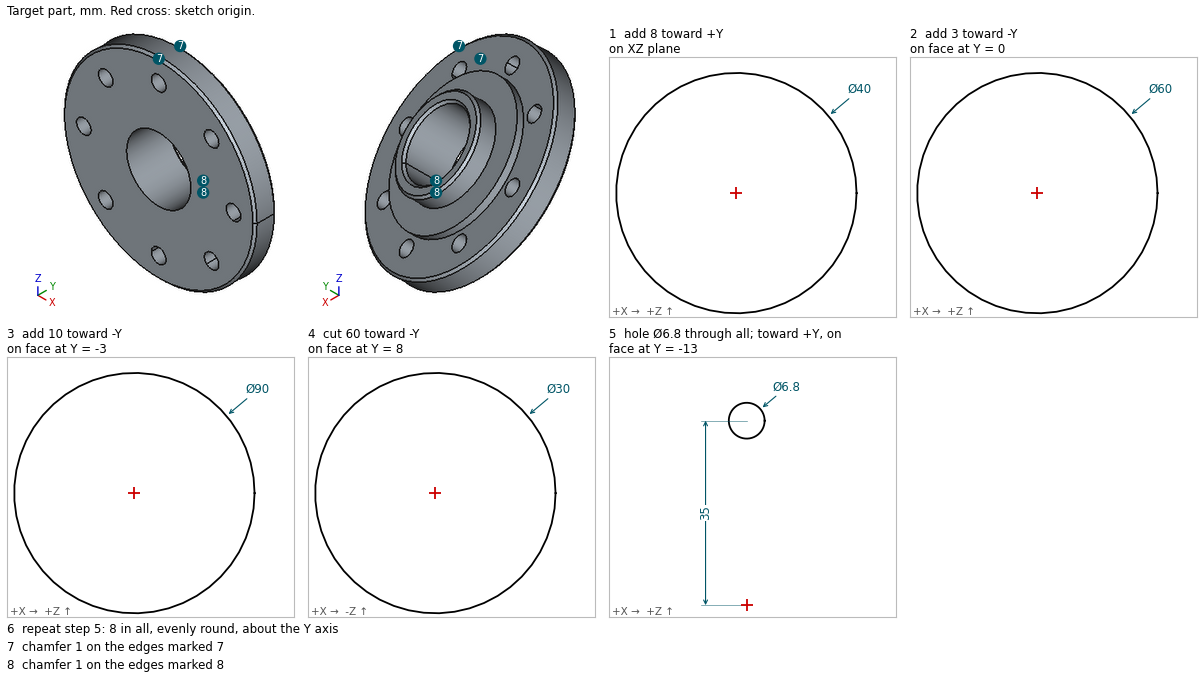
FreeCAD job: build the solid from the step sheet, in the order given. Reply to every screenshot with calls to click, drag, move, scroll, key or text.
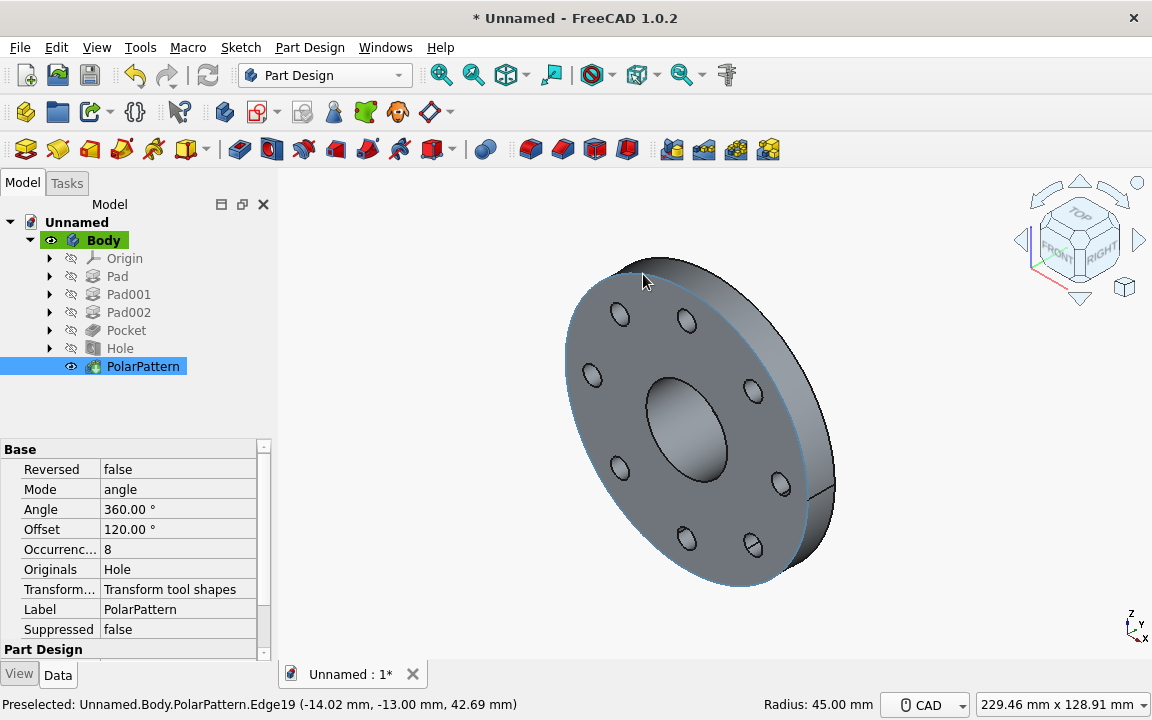
key(2)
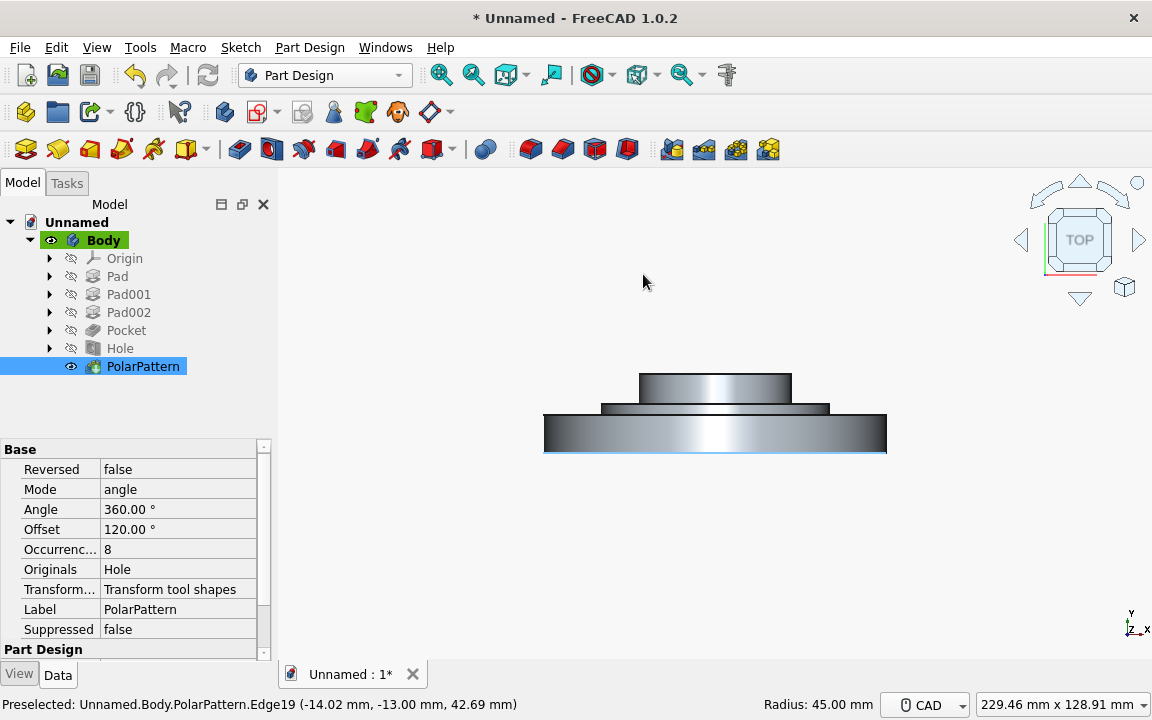
click(442, 76)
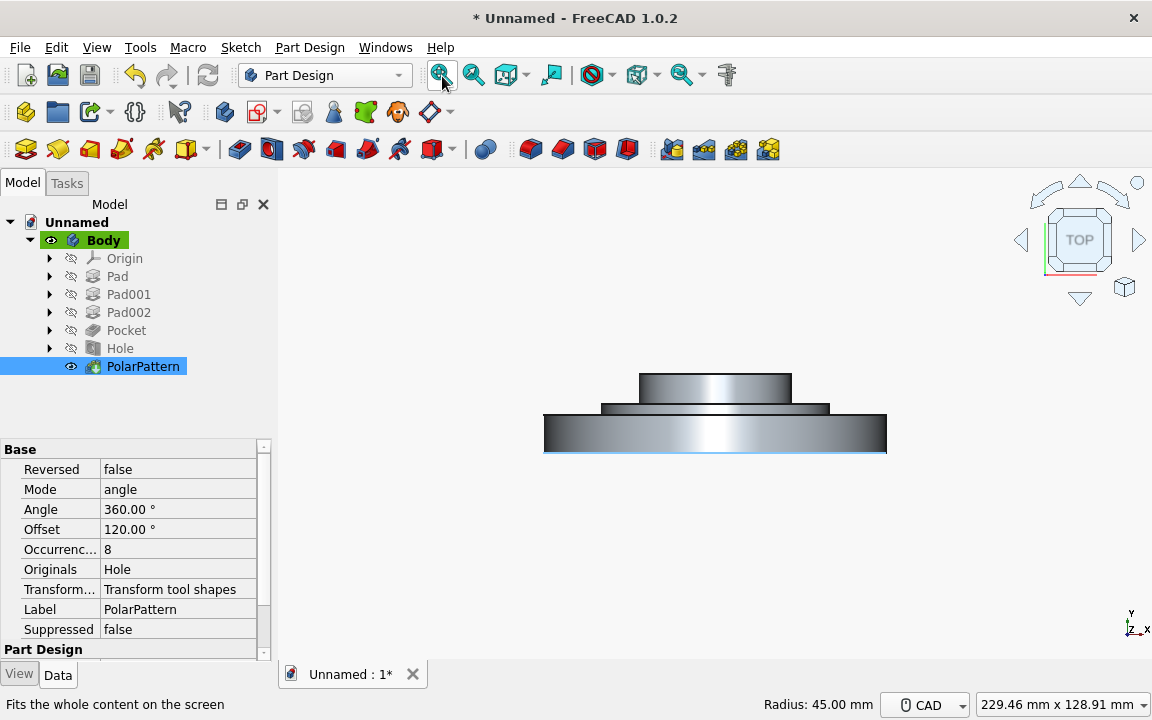
click(576, 414, ctrl)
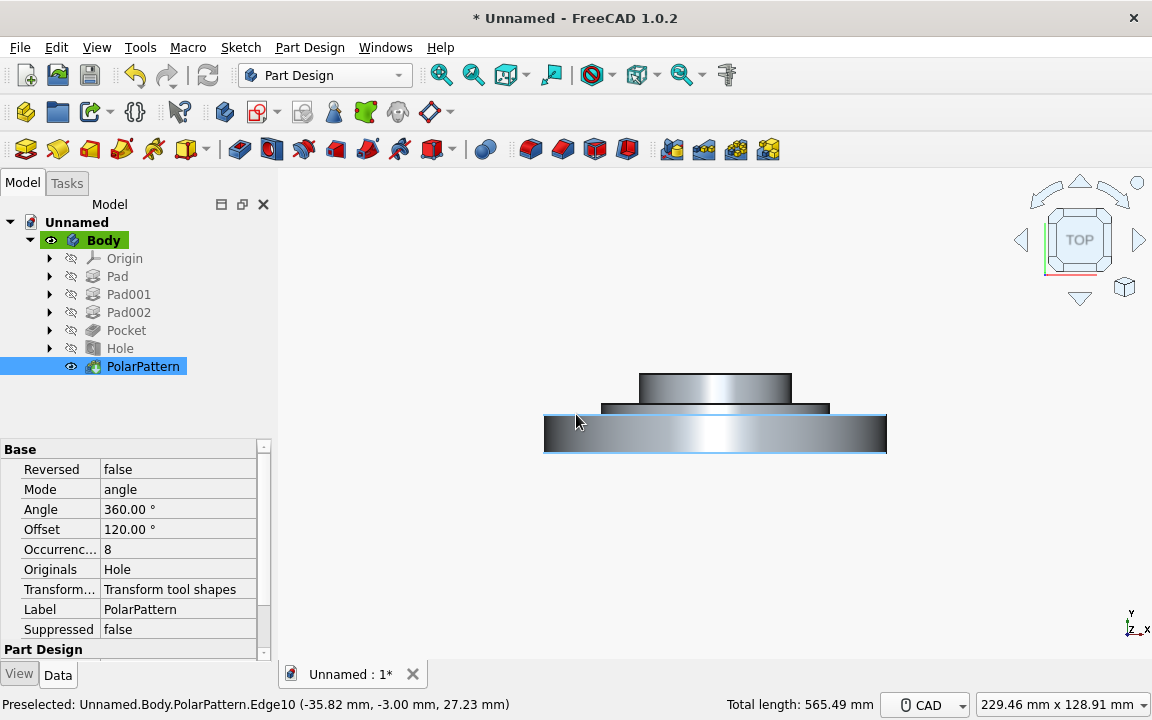
click(564, 150)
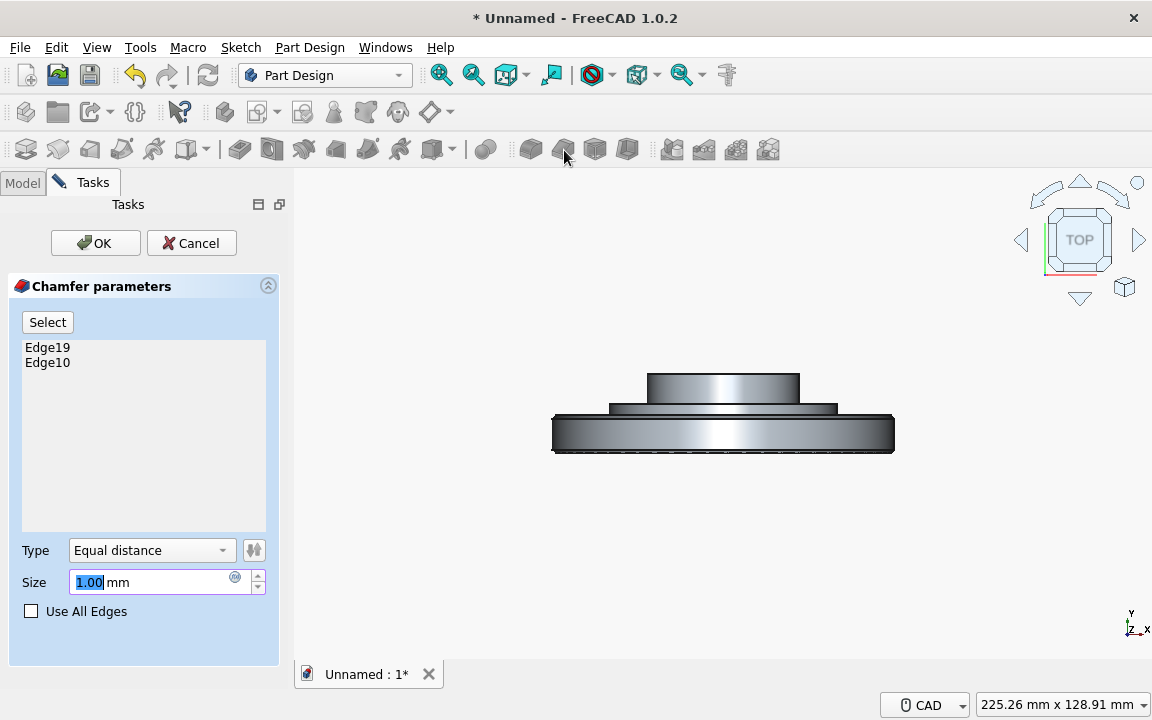
text(1)
key(Tab)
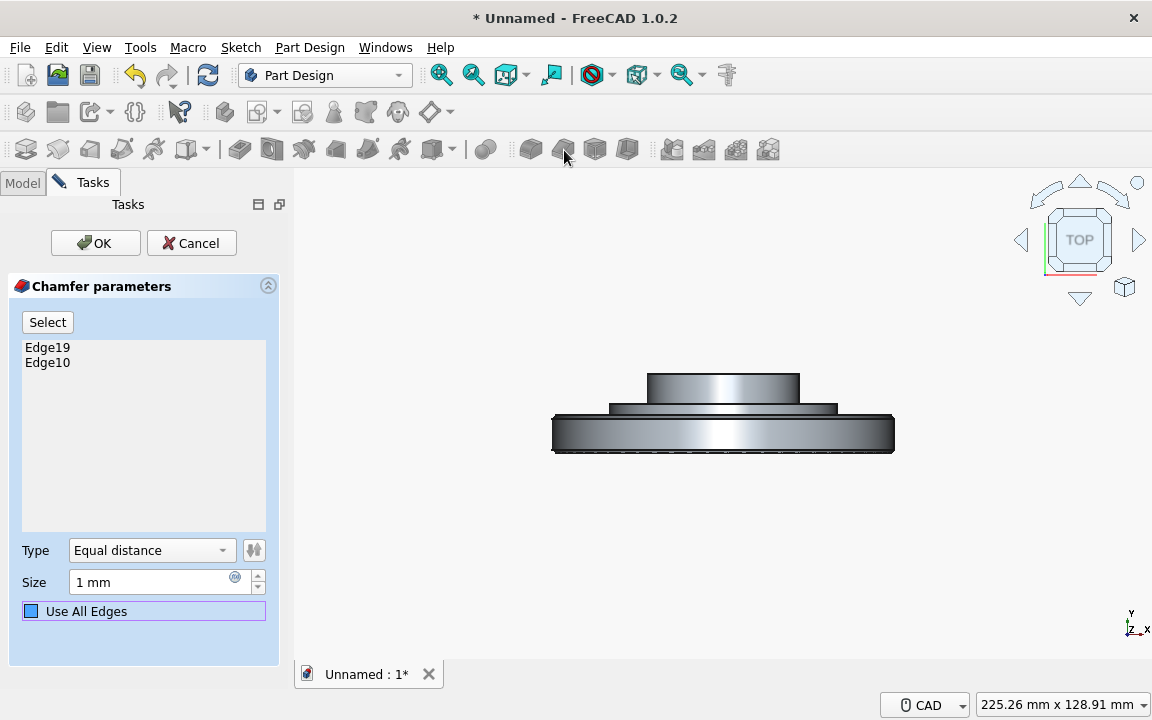
click(96, 243)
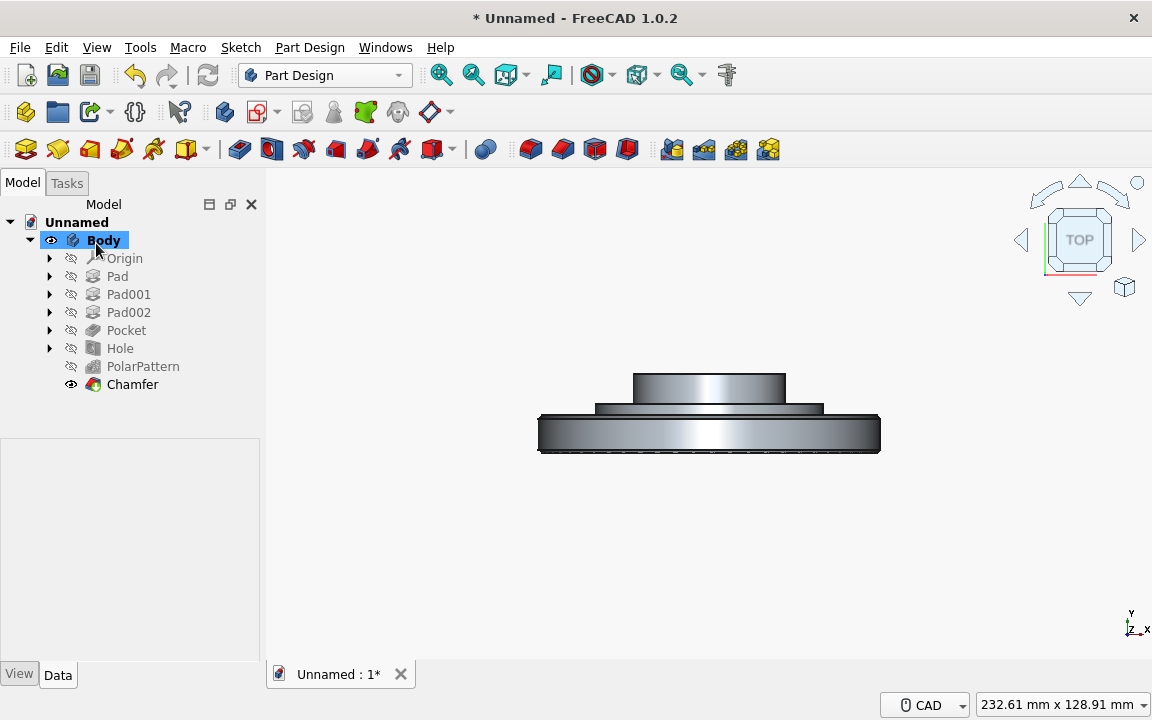
key(v)
key(f)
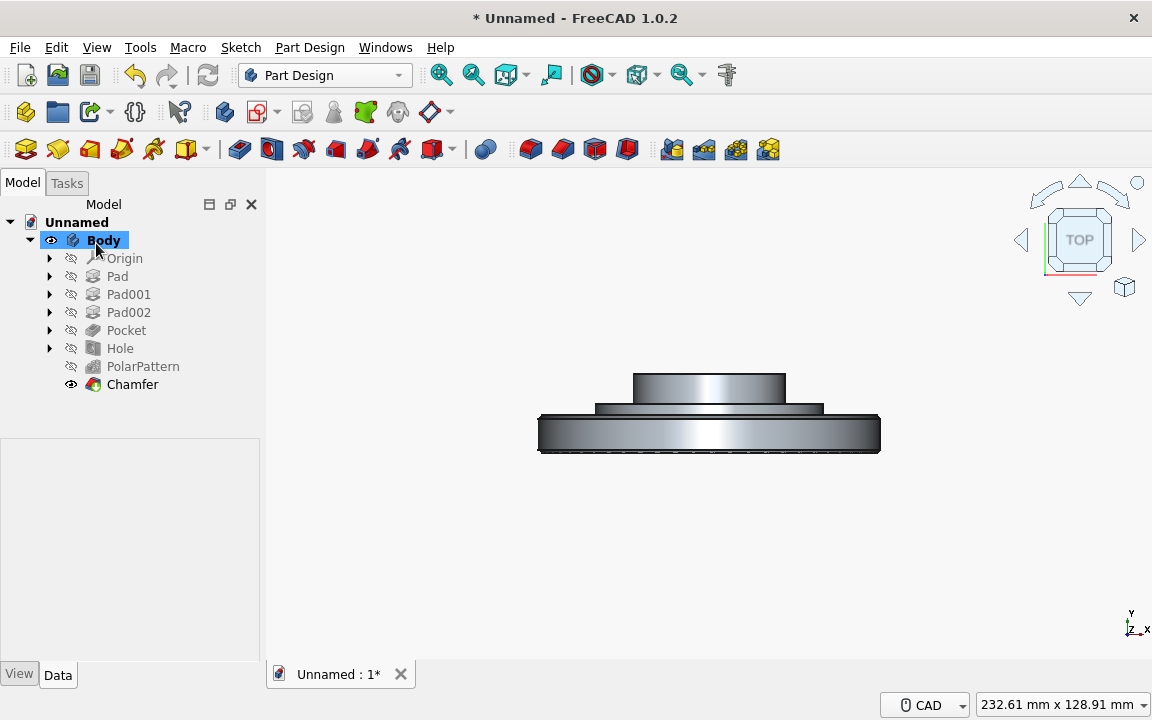
click(647, 373)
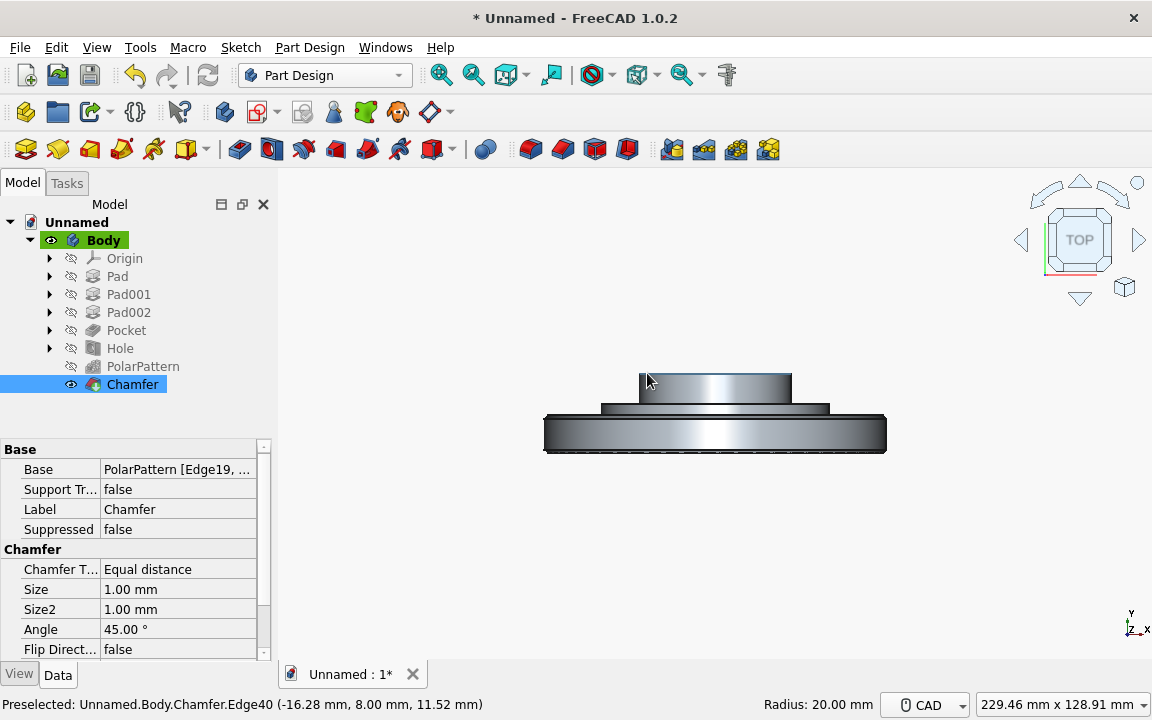
key(0)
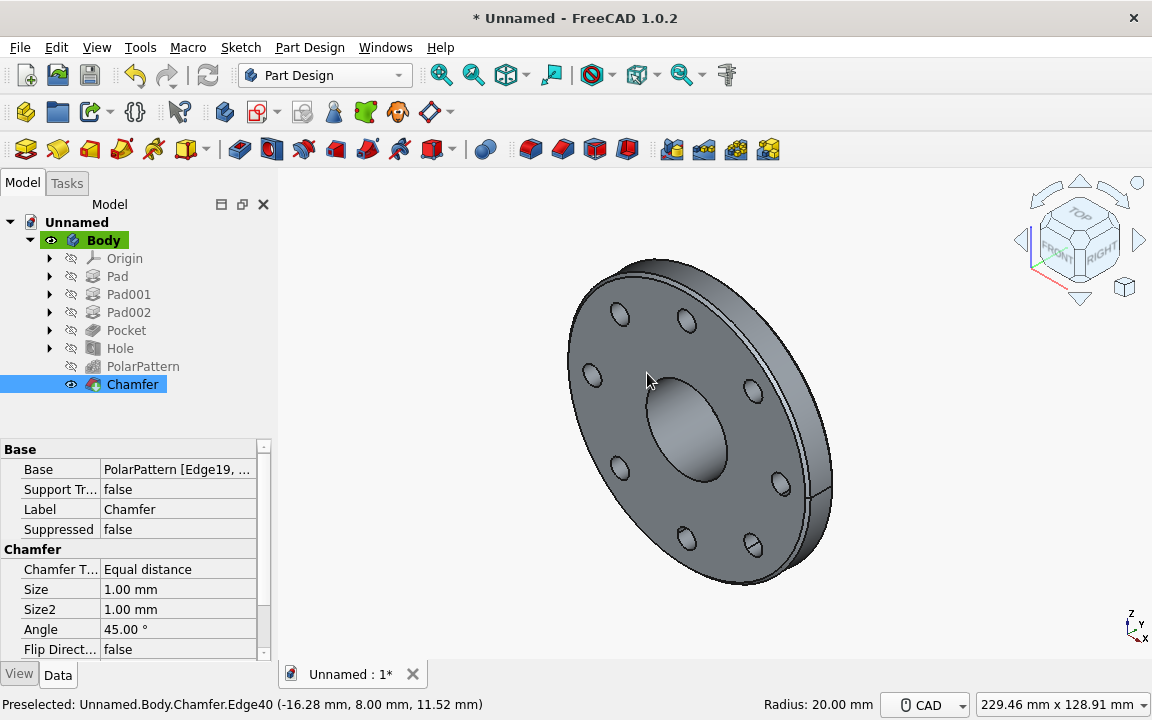
key(2)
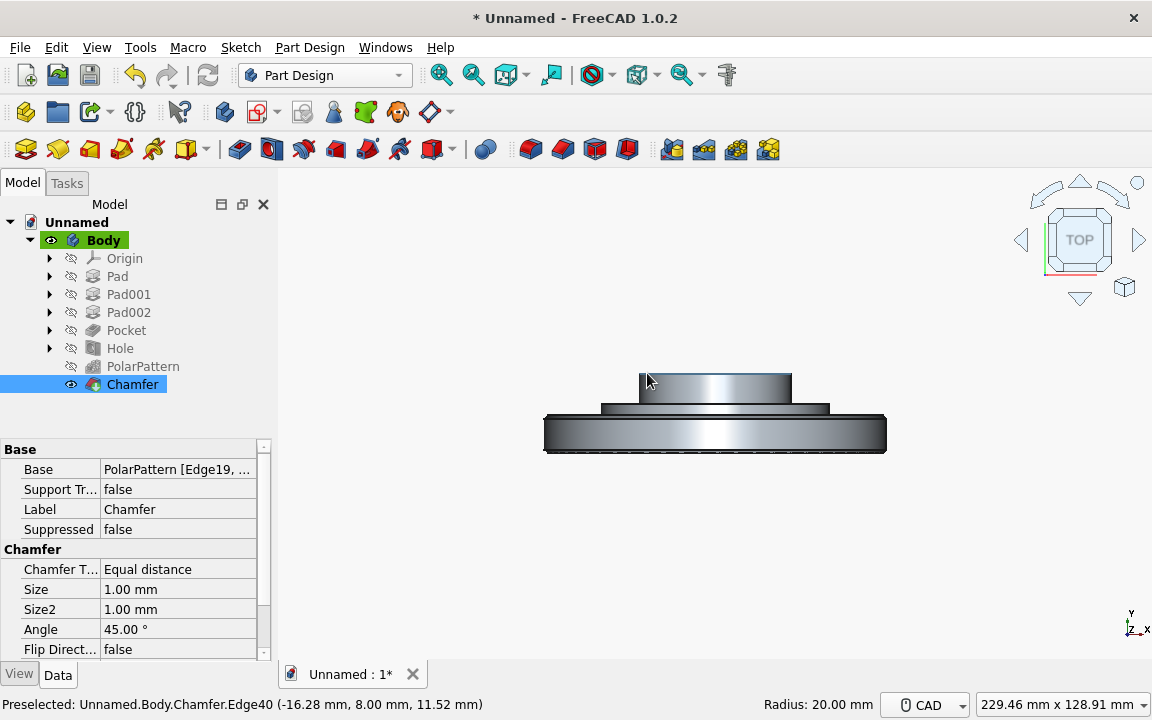
click(442, 76)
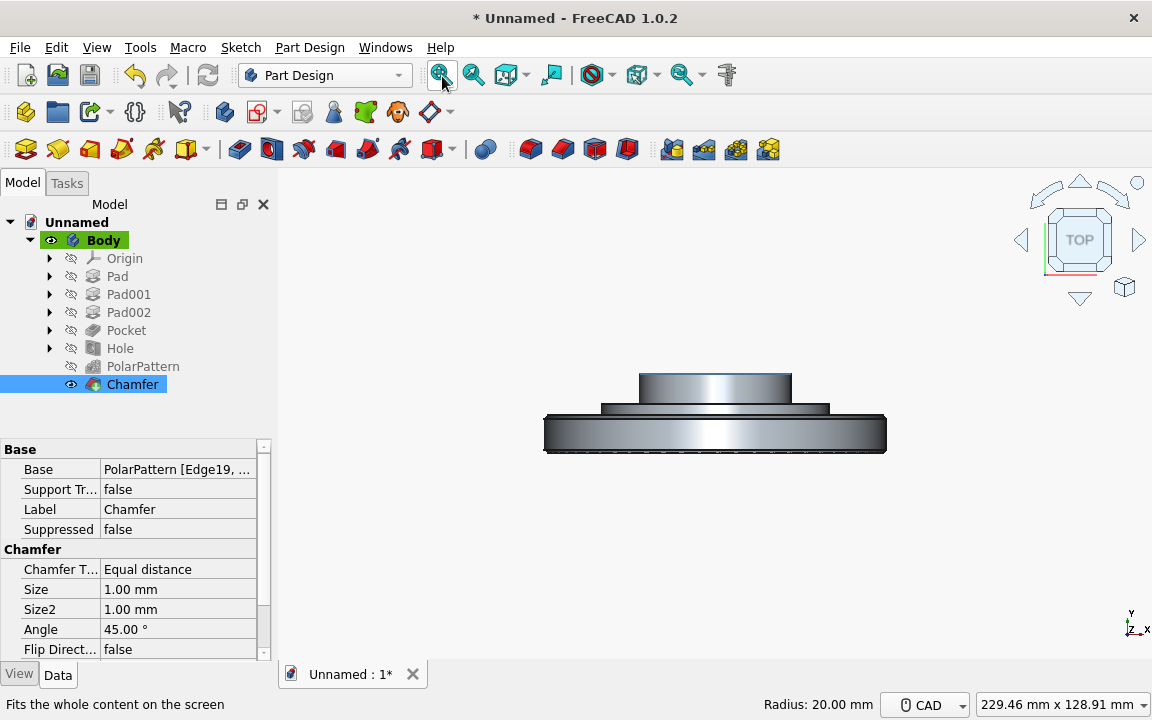
key(1)